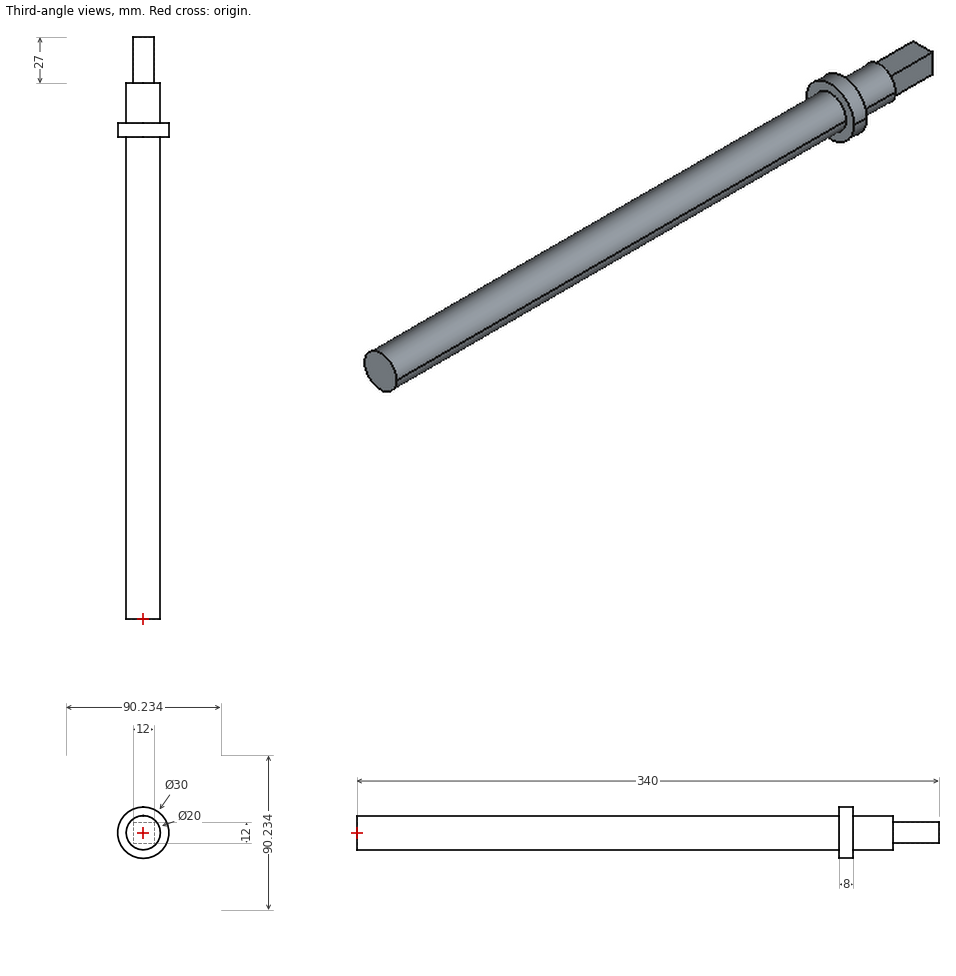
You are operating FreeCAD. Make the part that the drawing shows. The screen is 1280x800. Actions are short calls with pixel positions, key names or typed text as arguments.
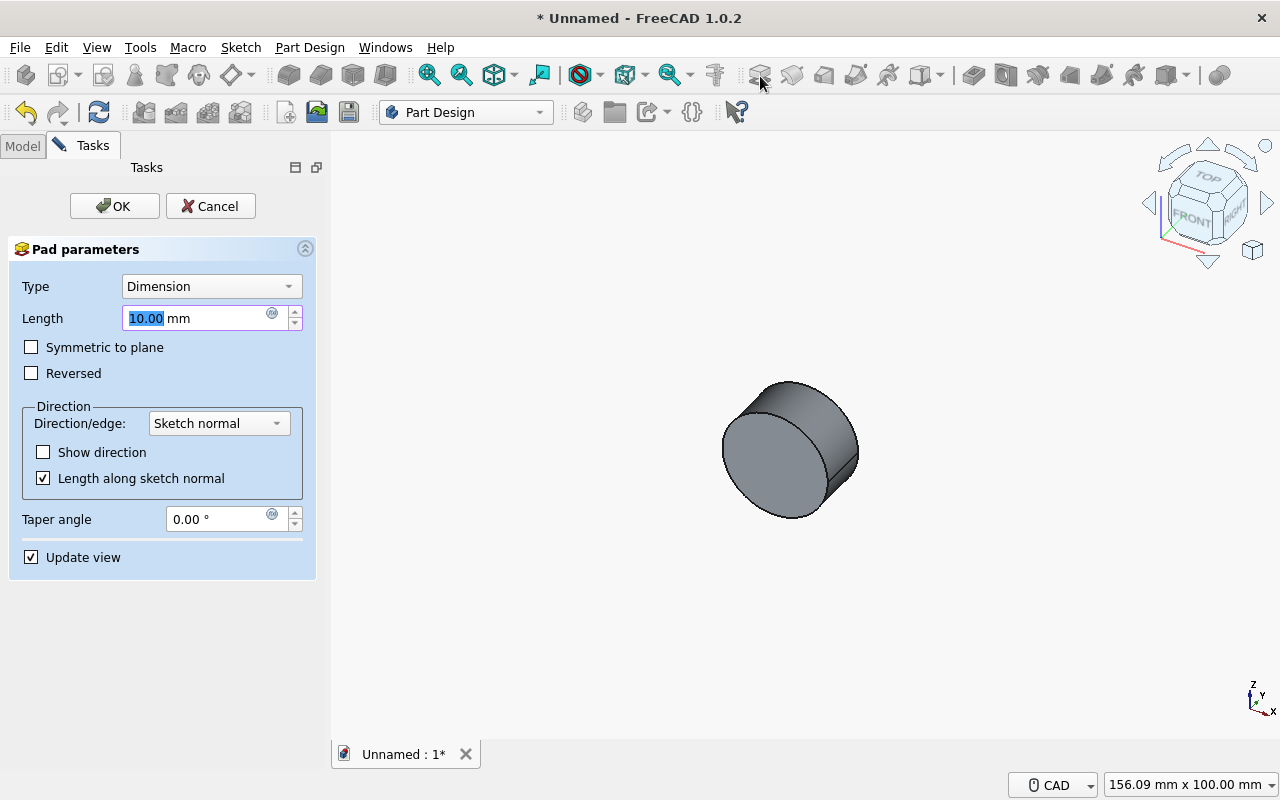
text(340)
key(Tab)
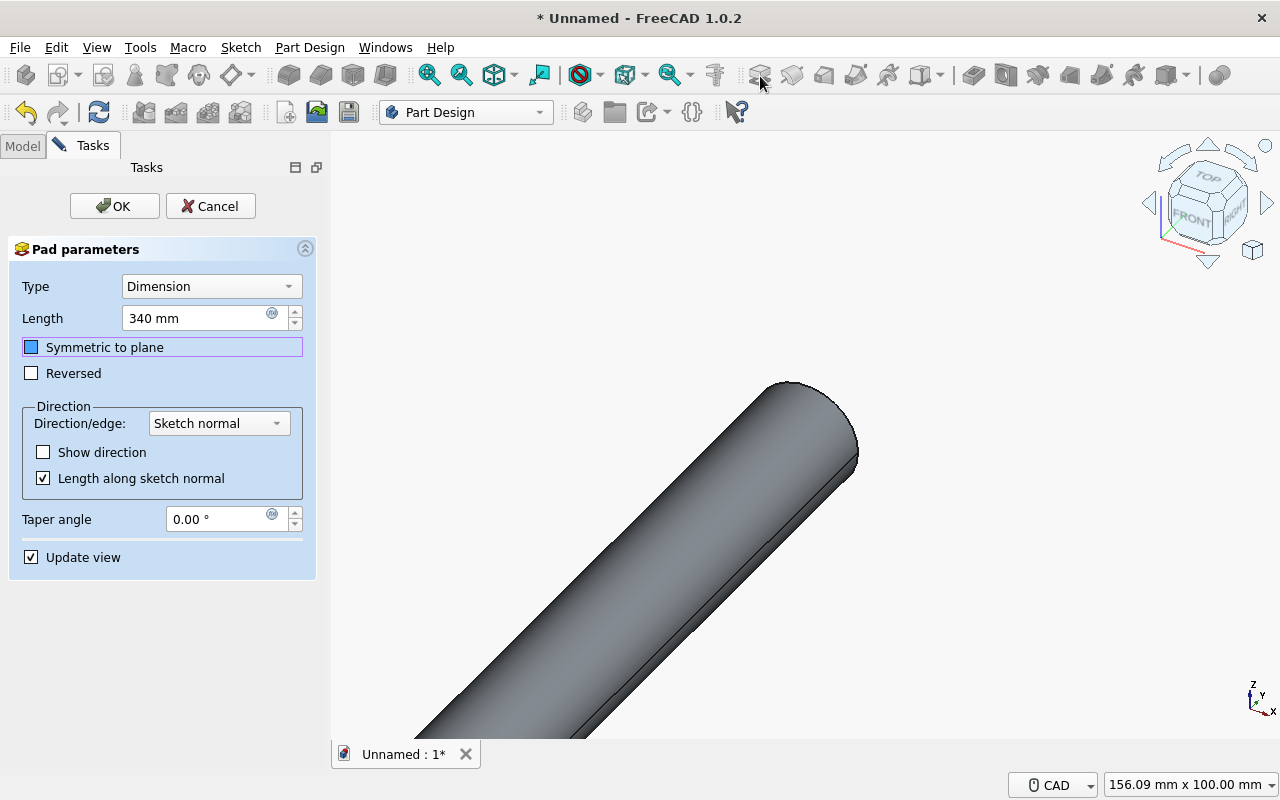
click(30, 373)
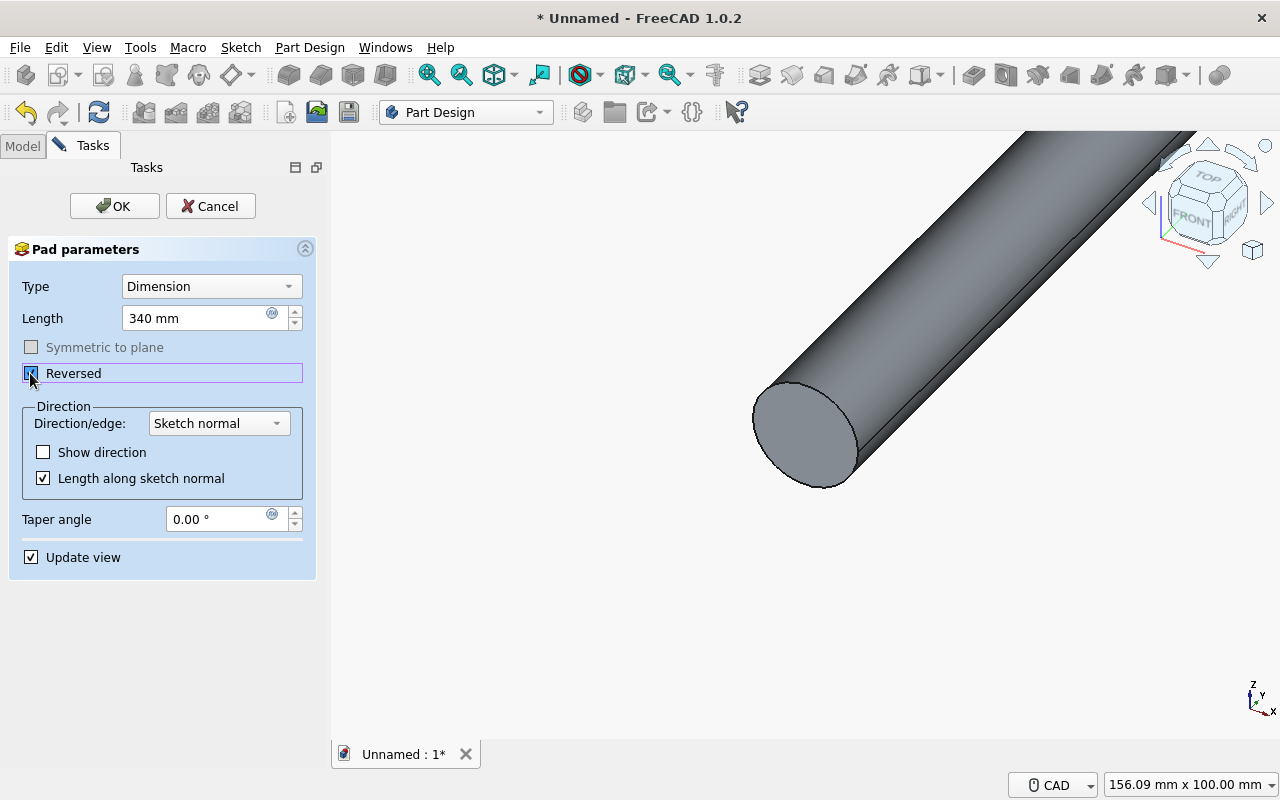
click(115, 206)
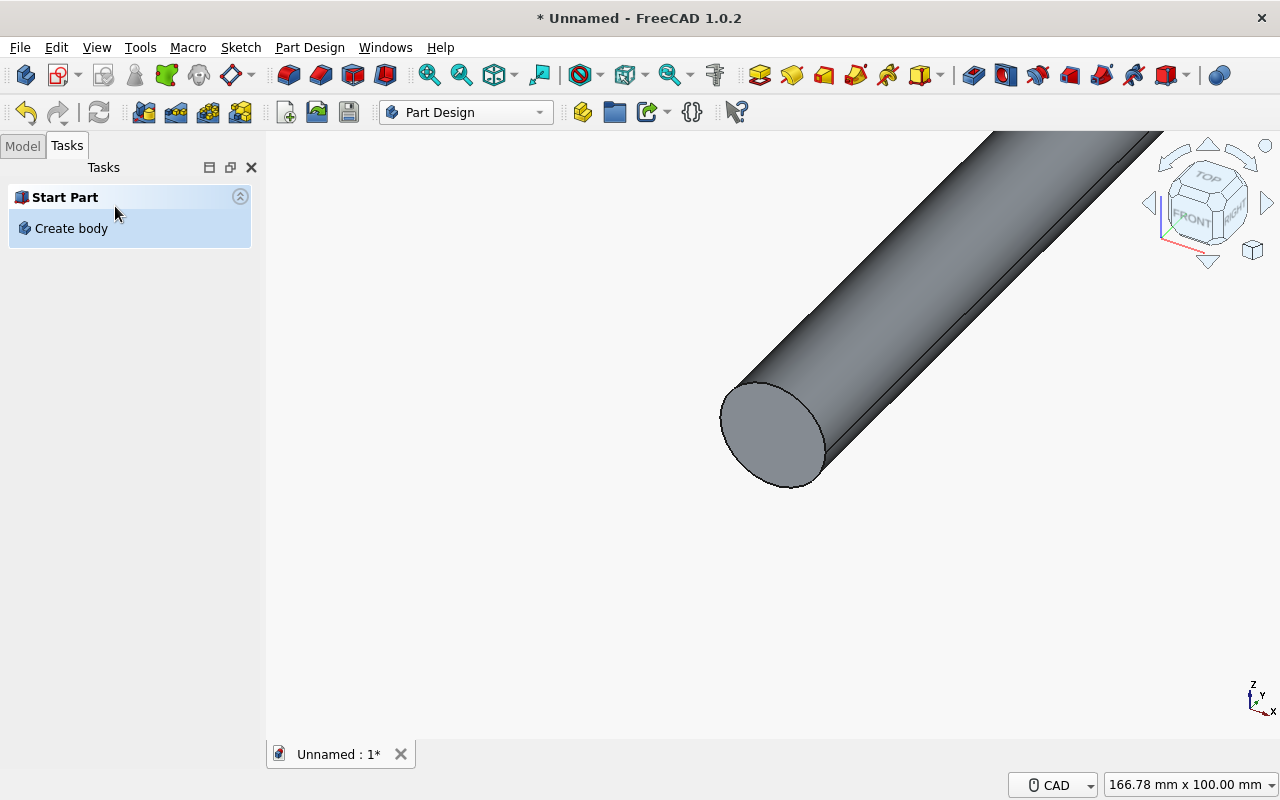
key(v)
key(f)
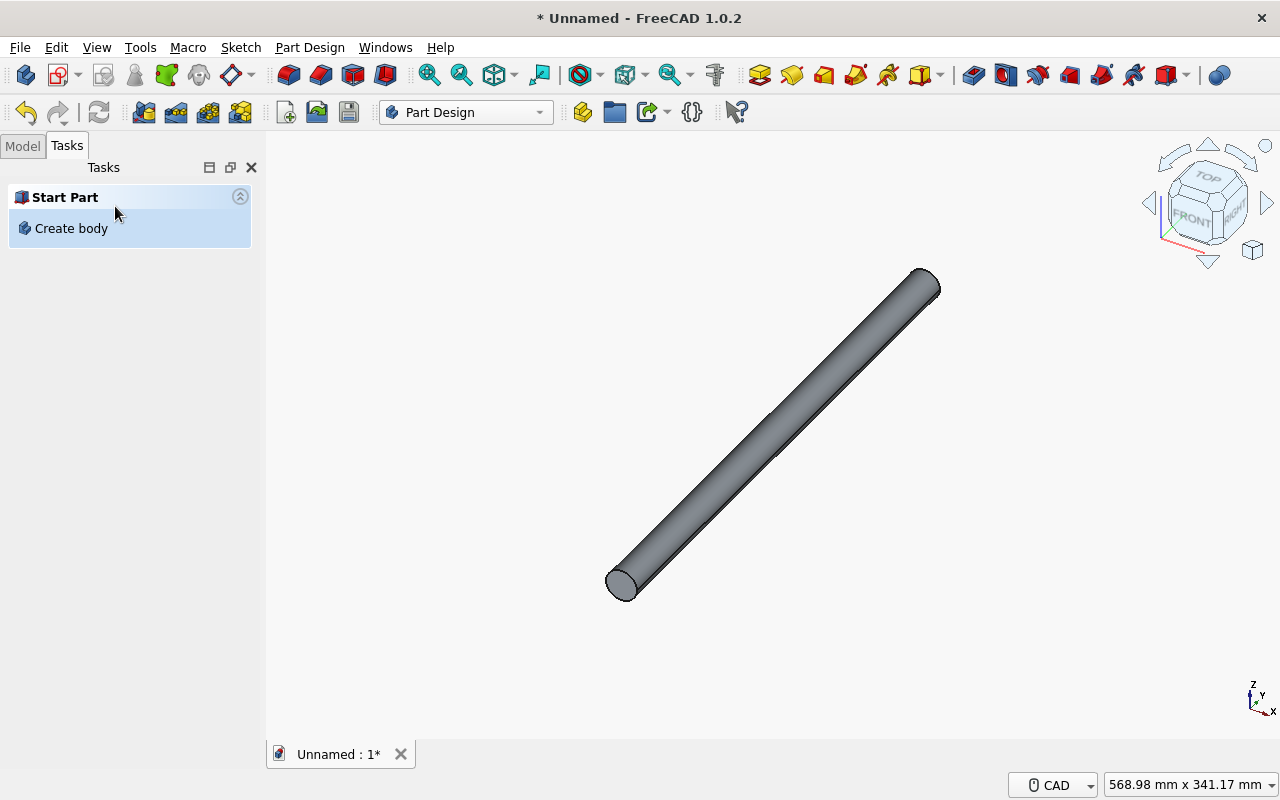
key(4)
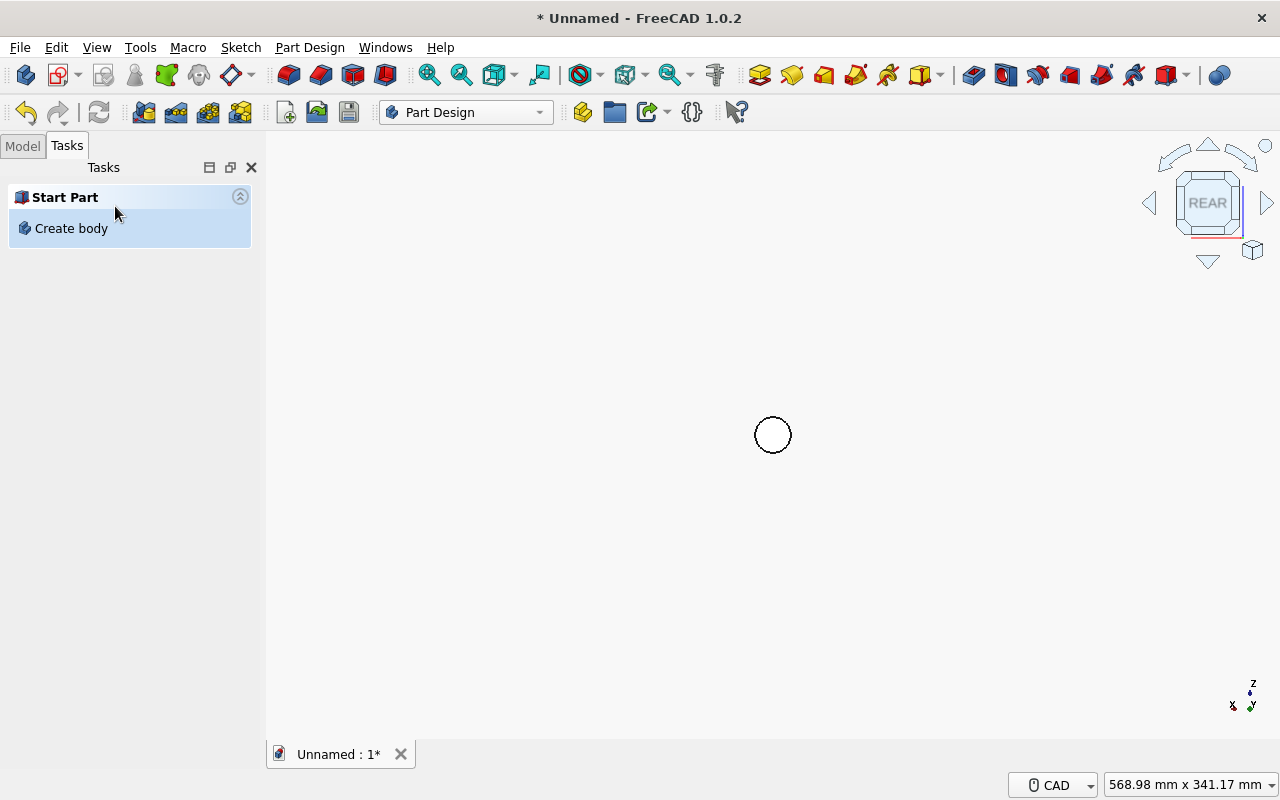
key(v)
key(f)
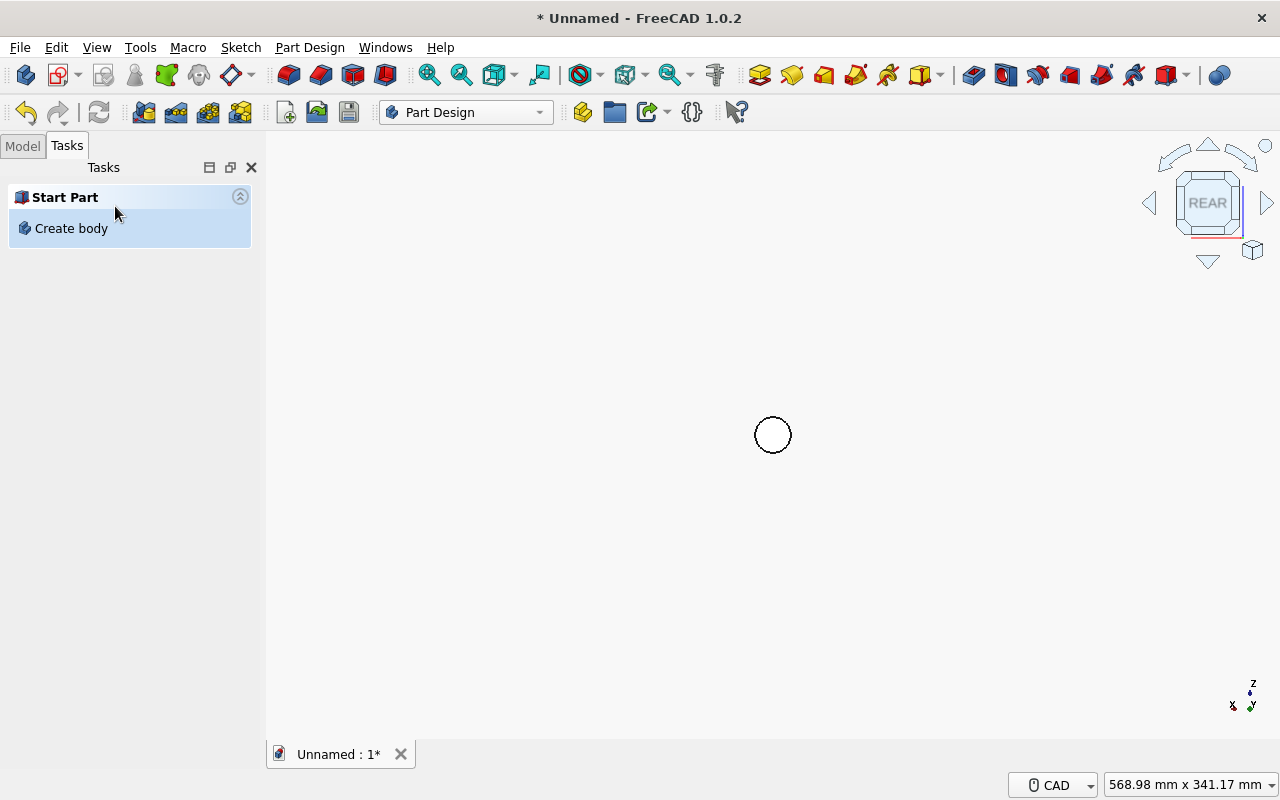
click(773, 434)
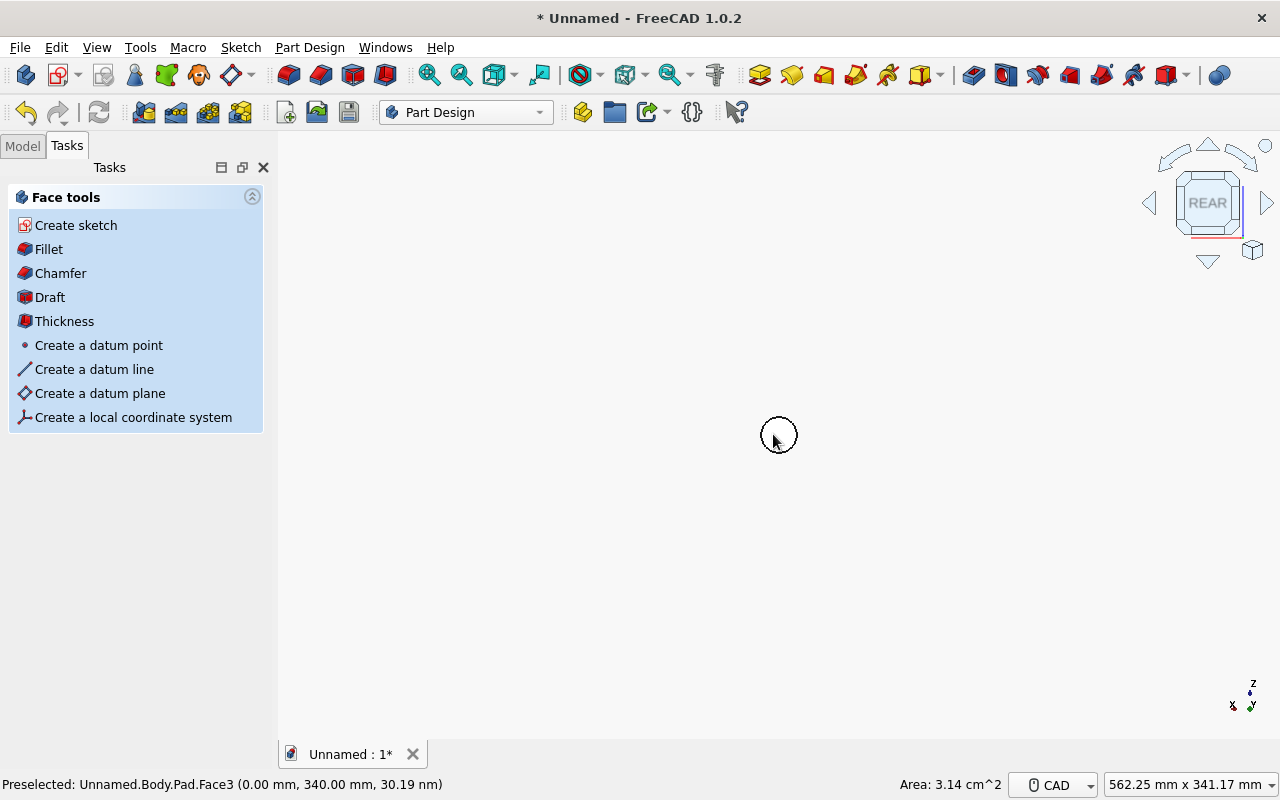
click(58, 76)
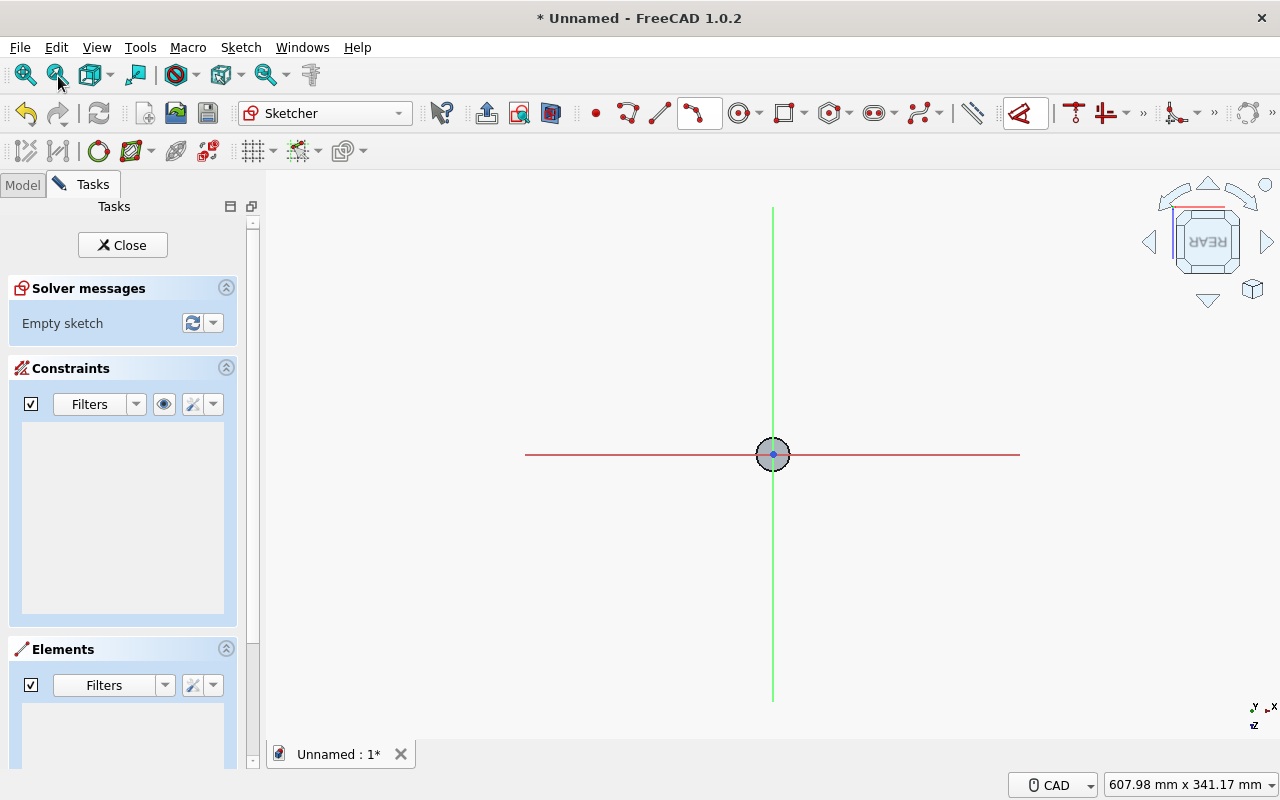
scroll(829, 454, up, 4)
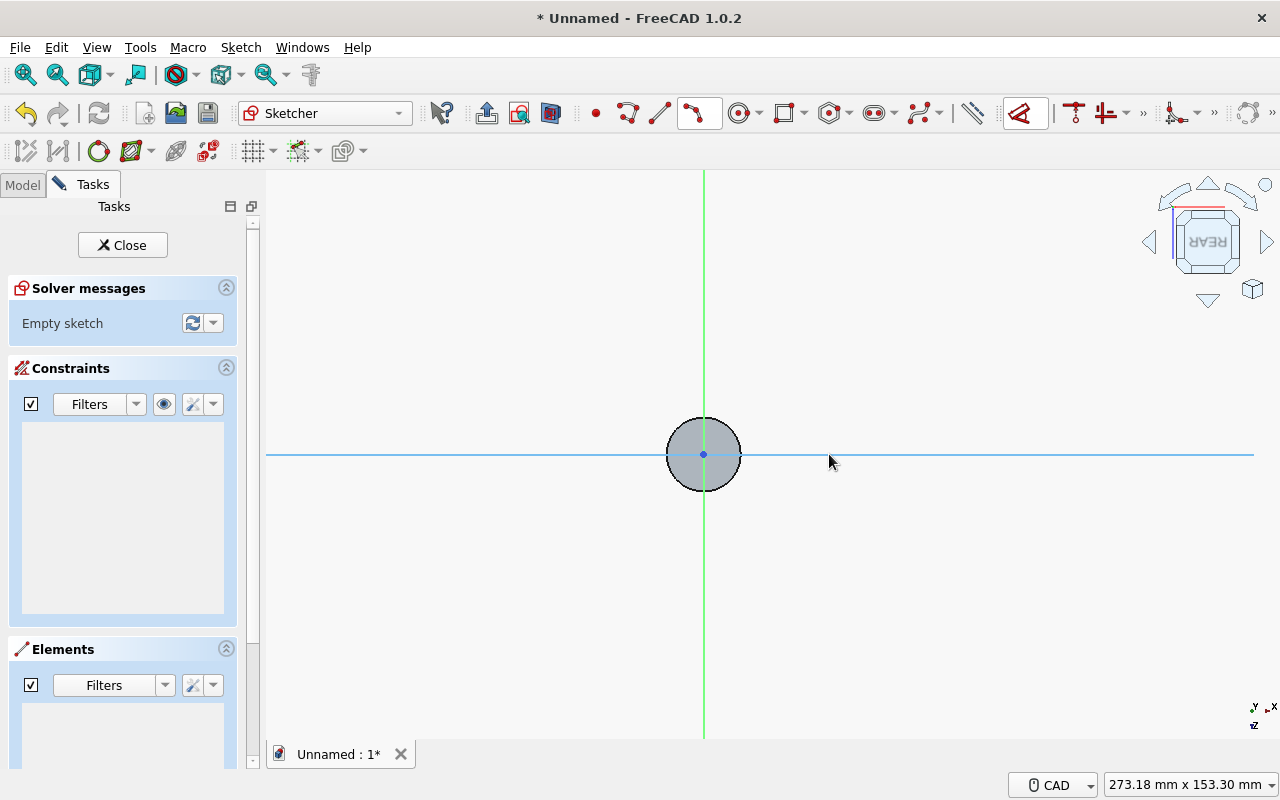
key(g)
key(v)